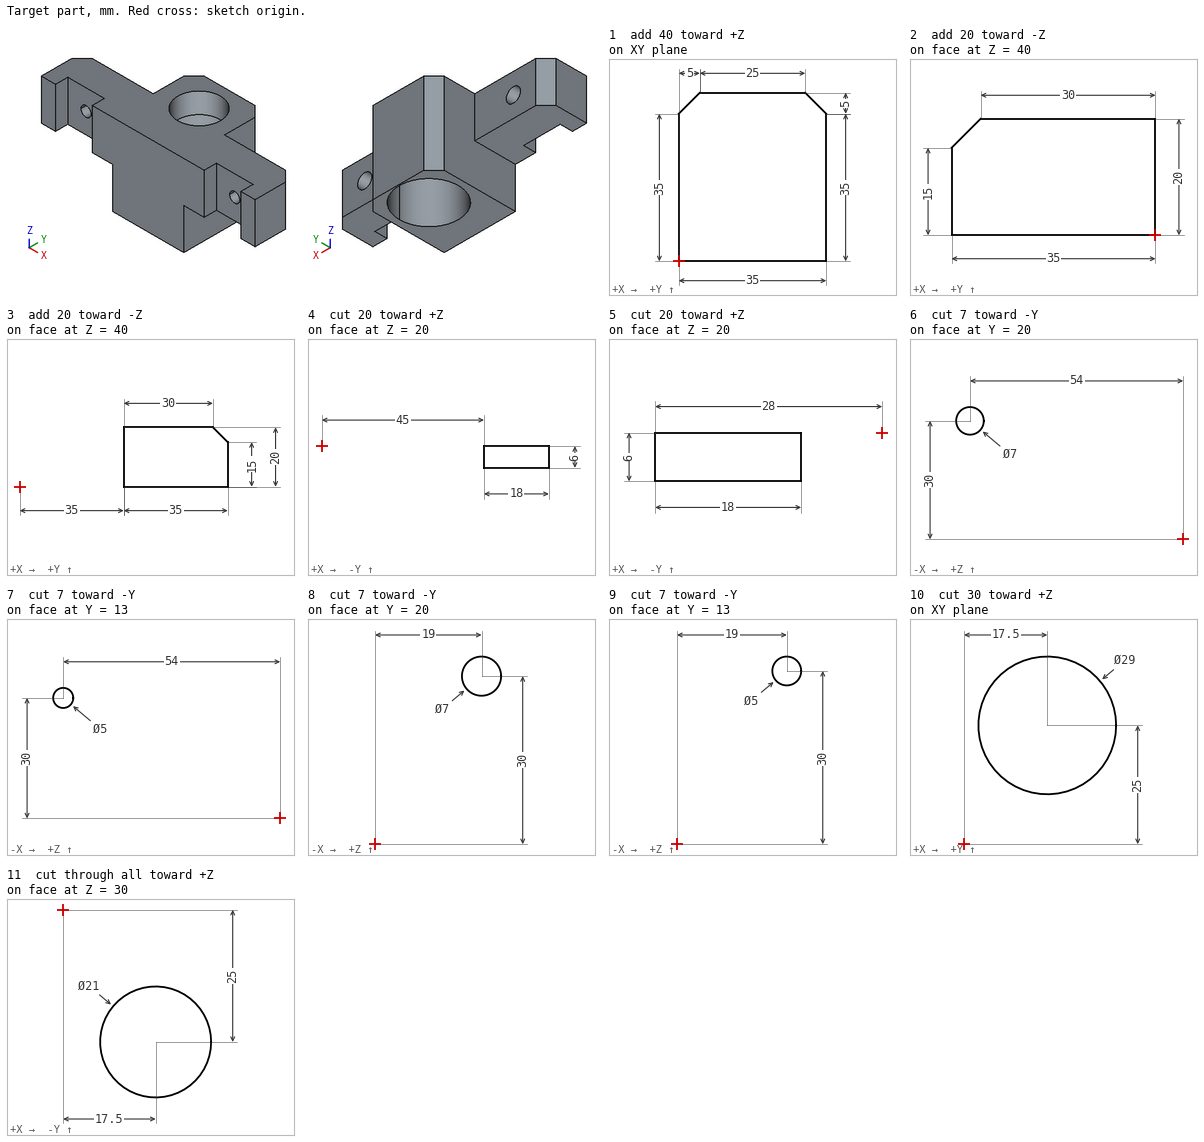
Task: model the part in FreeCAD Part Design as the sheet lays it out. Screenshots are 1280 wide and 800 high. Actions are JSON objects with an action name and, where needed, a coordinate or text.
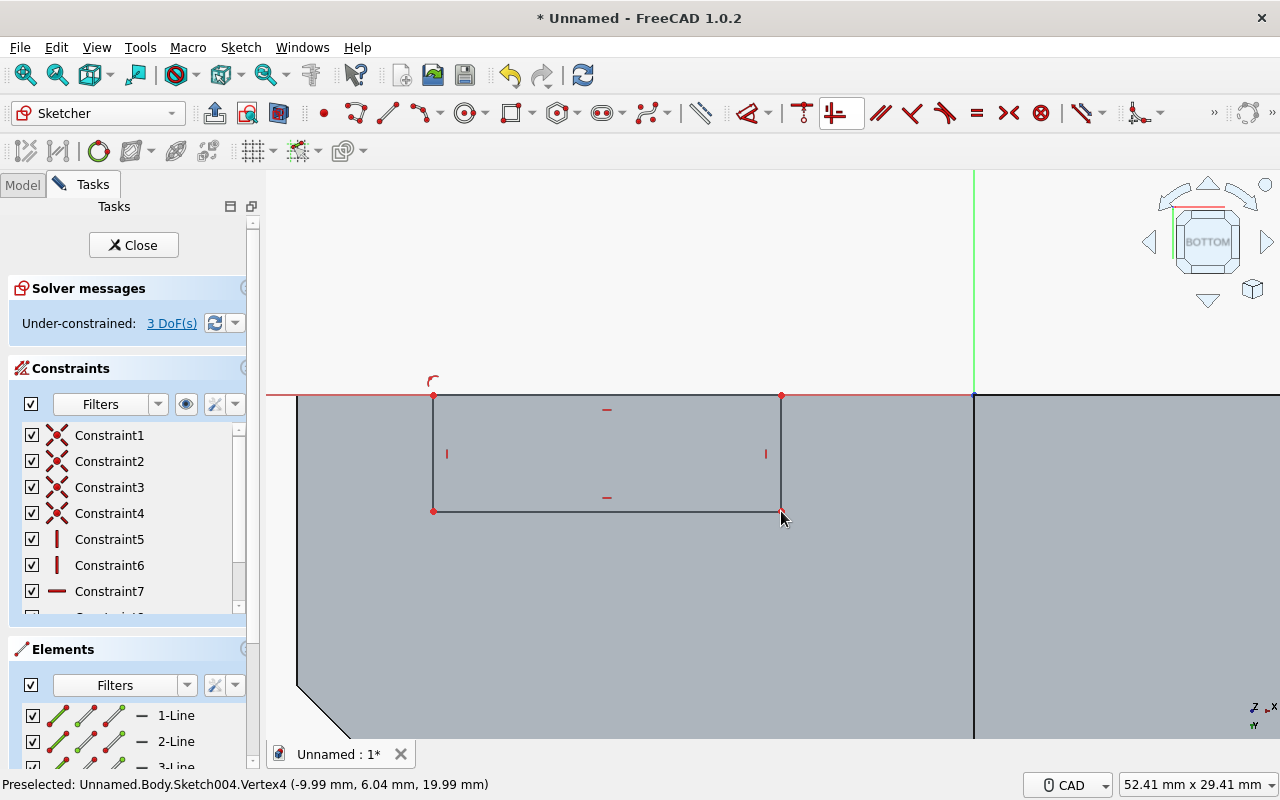
{"action": "left_click", "coordinate": [748, 114]}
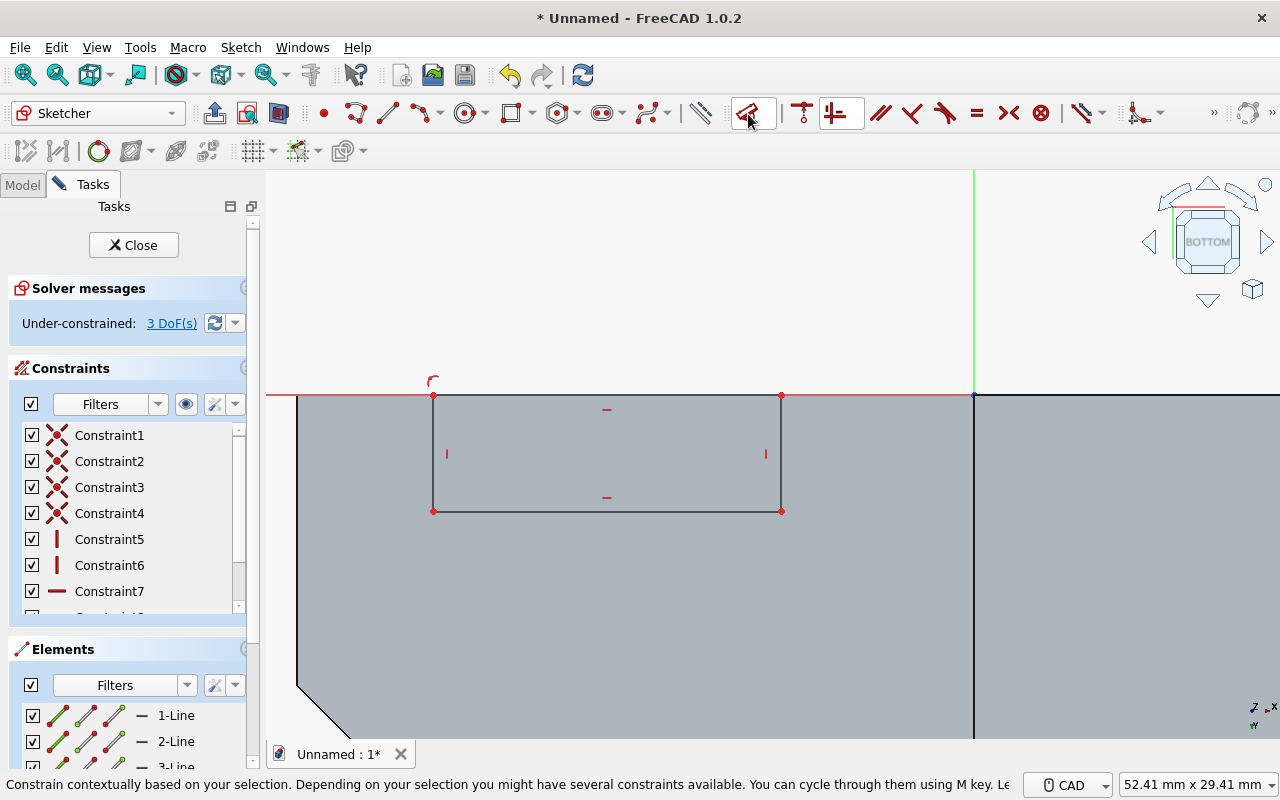
{"action": "left_click", "coordinate": [433, 430]}
{"action": "left_click", "coordinate": [399, 454]}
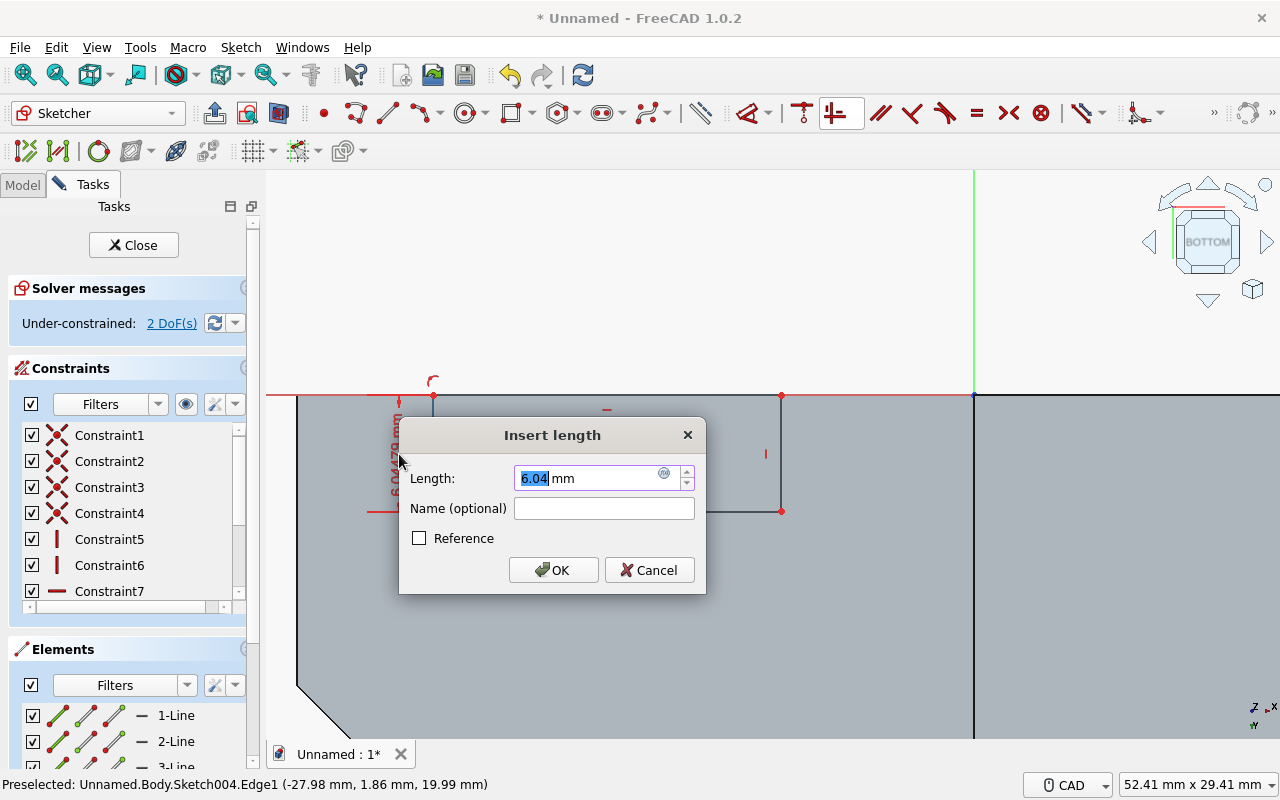
{"action": "type", "text": "6"}
{"action": "key", "text": "Return"}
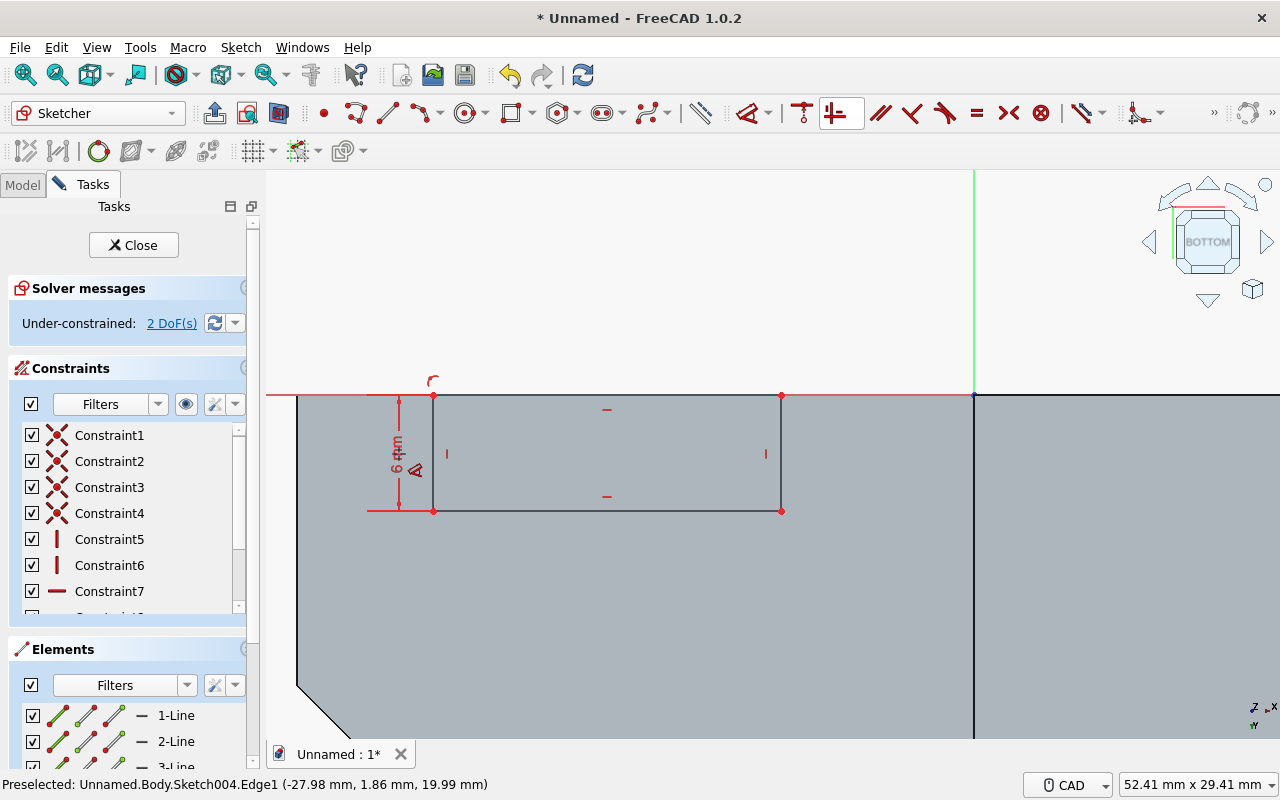
{"action": "left_click", "coordinate": [537, 511]}
{"action": "left_click", "coordinate": [607, 545]}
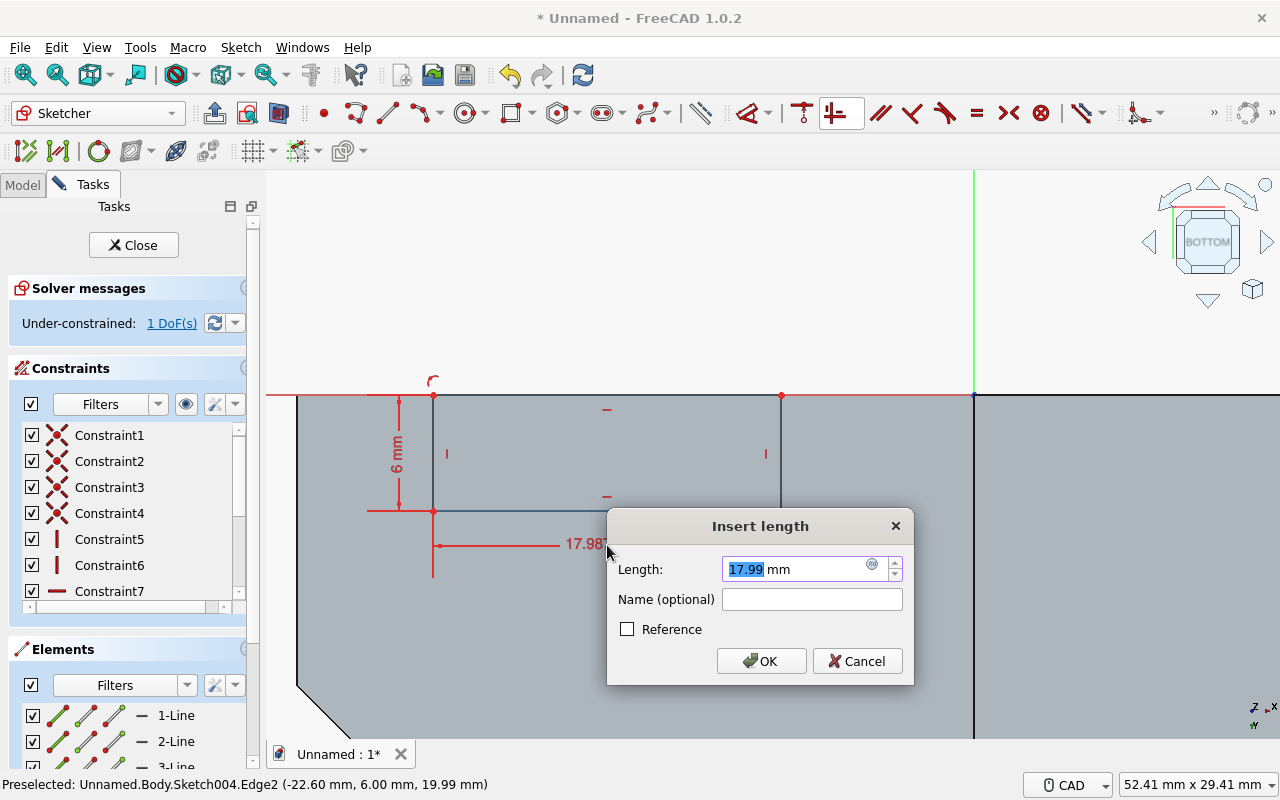
{"action": "type", "text": "18"}
{"action": "key", "text": "Return"}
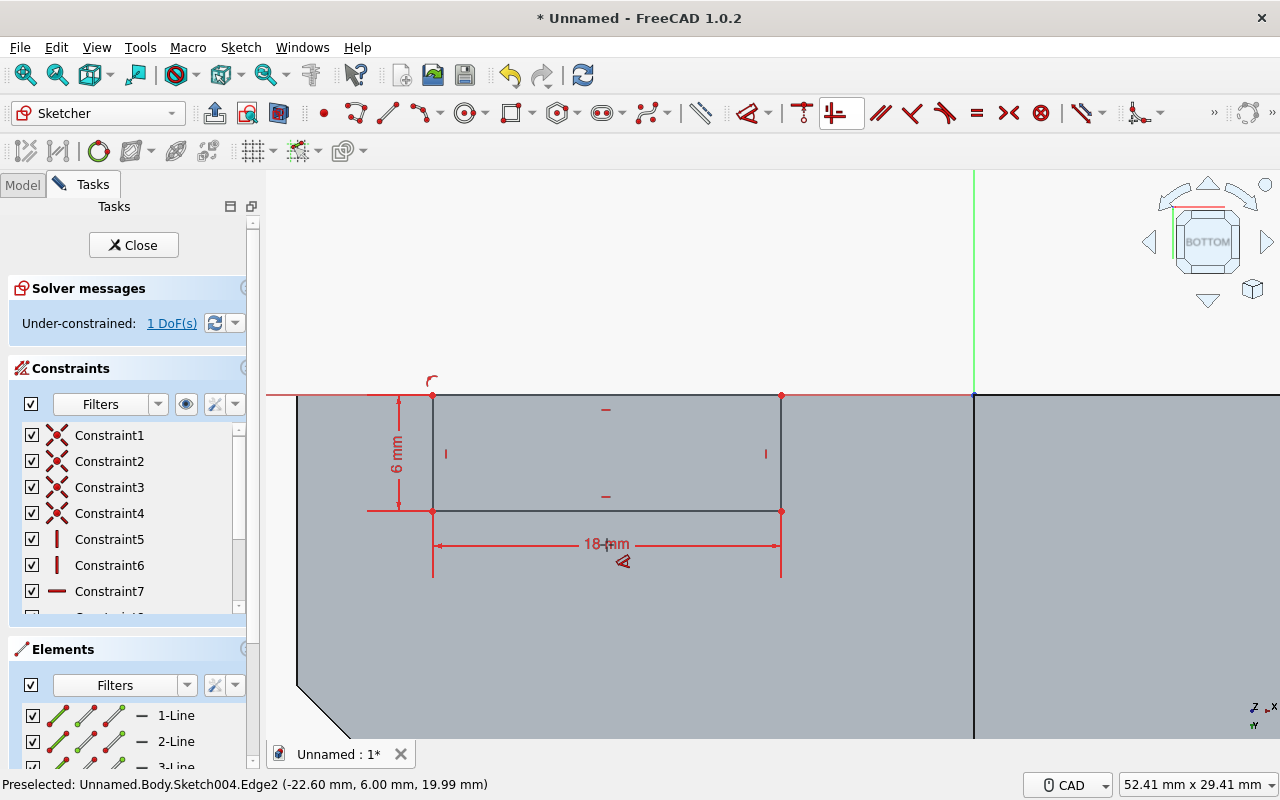
{"action": "left_click", "coordinate": [433, 395]}
{"action": "left_click", "coordinate": [703, 361]}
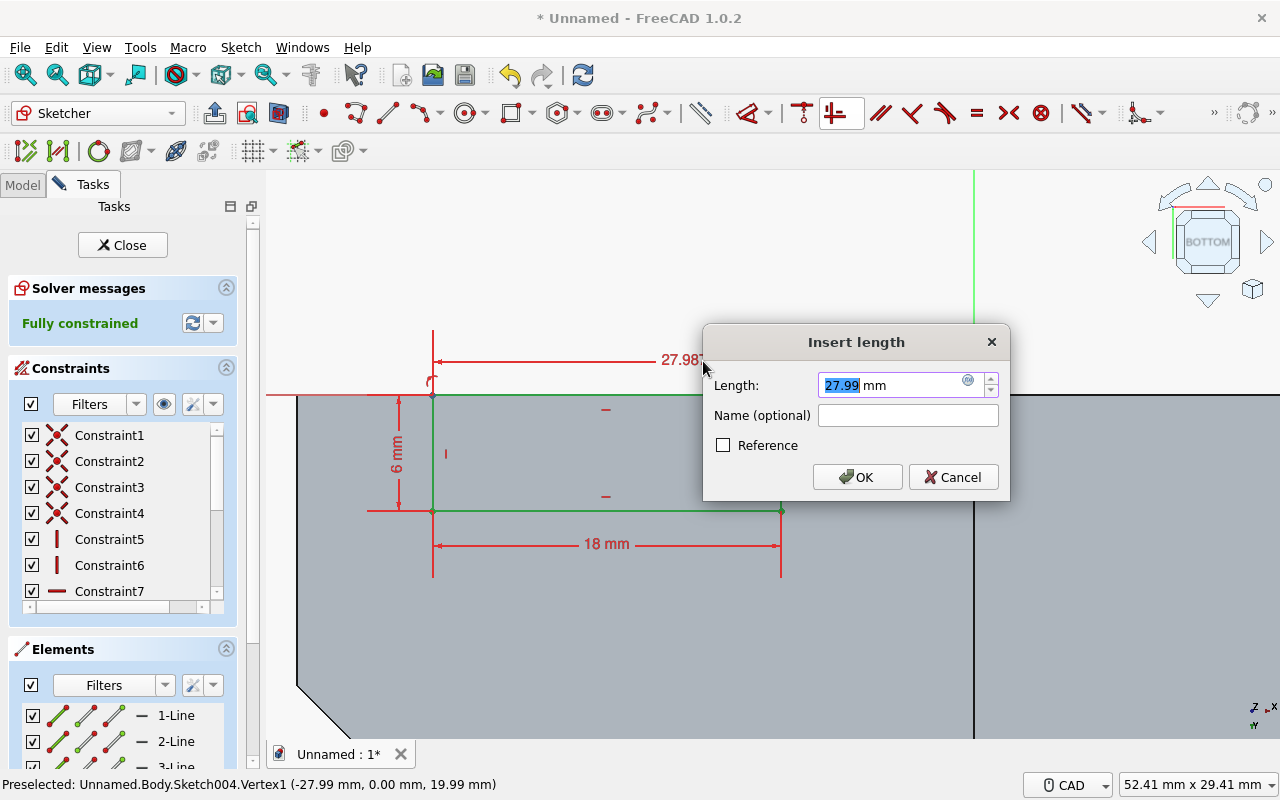
{"action": "type", "text": "28"}
{"action": "key", "text": "Return"}
{"action": "key", "text": "Escape"}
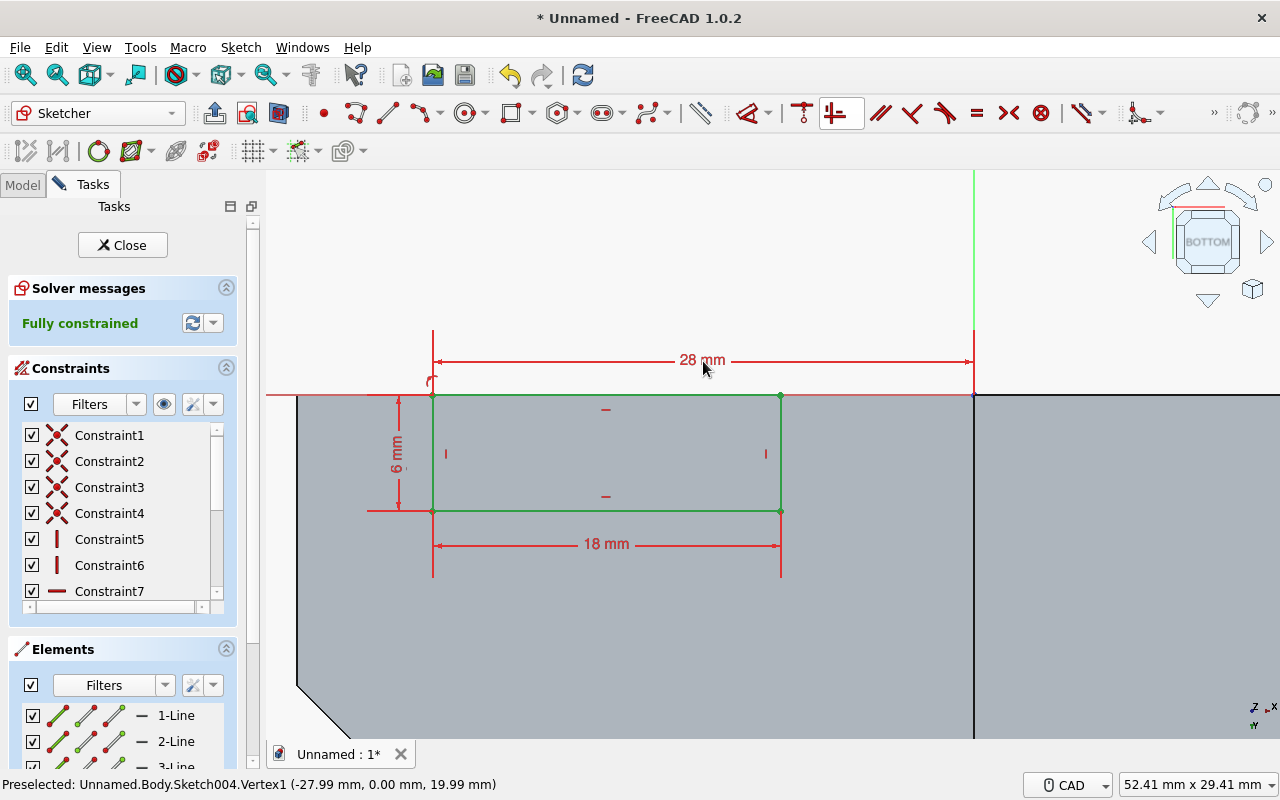
{"action": "left_click", "coordinate": [123, 245]}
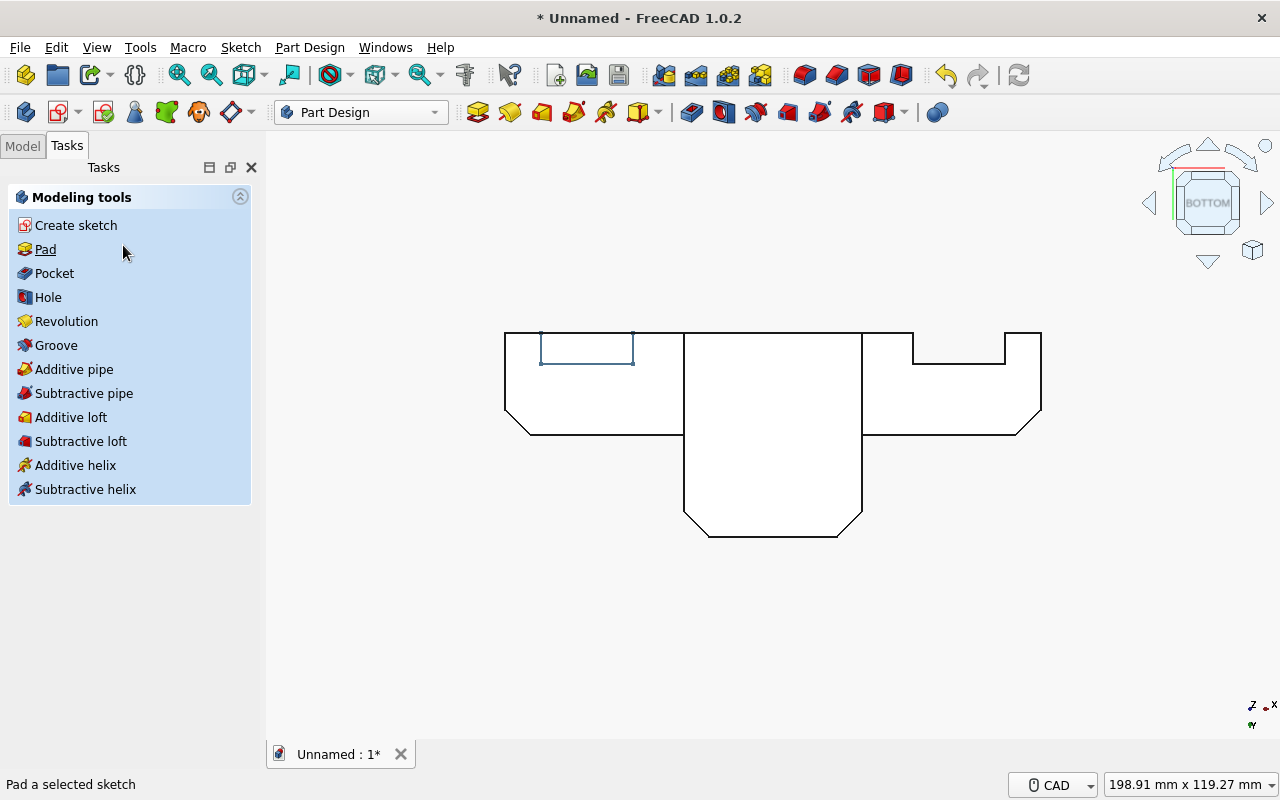
{"action": "left_click", "coordinate": [692, 112]}